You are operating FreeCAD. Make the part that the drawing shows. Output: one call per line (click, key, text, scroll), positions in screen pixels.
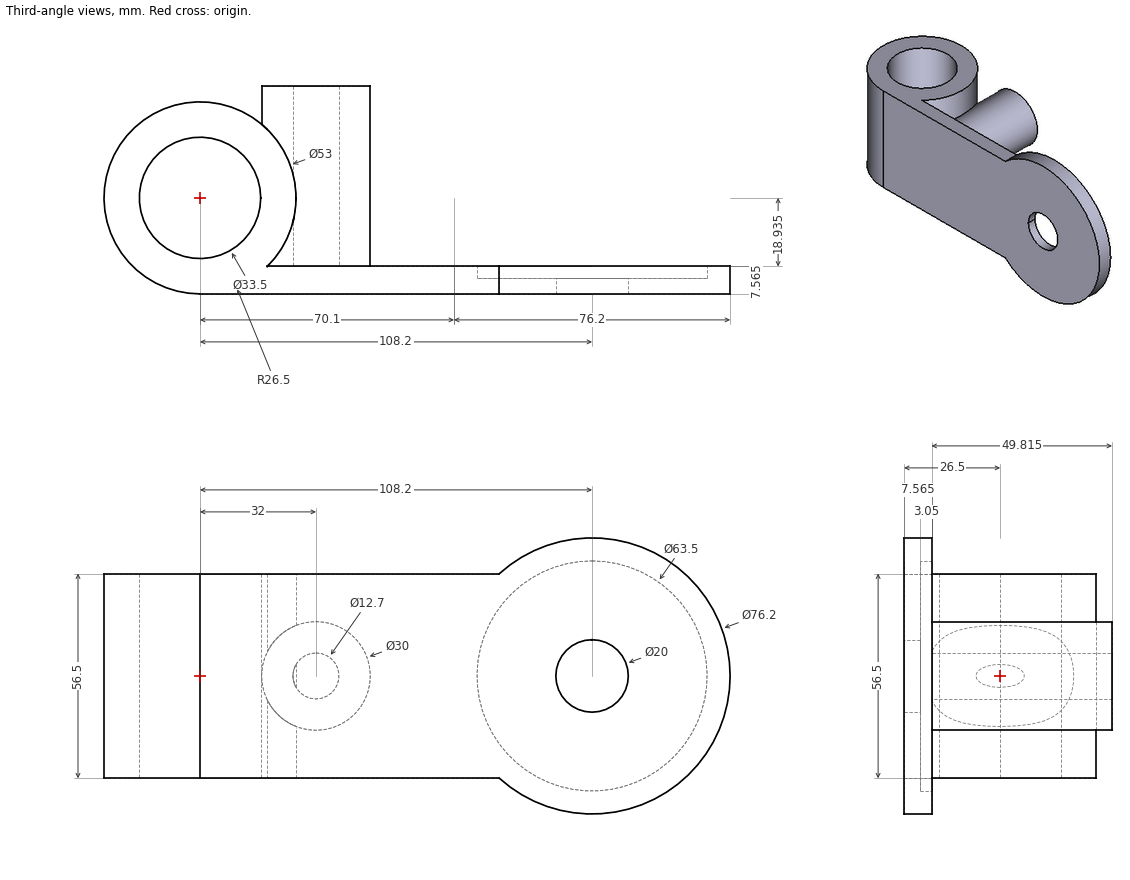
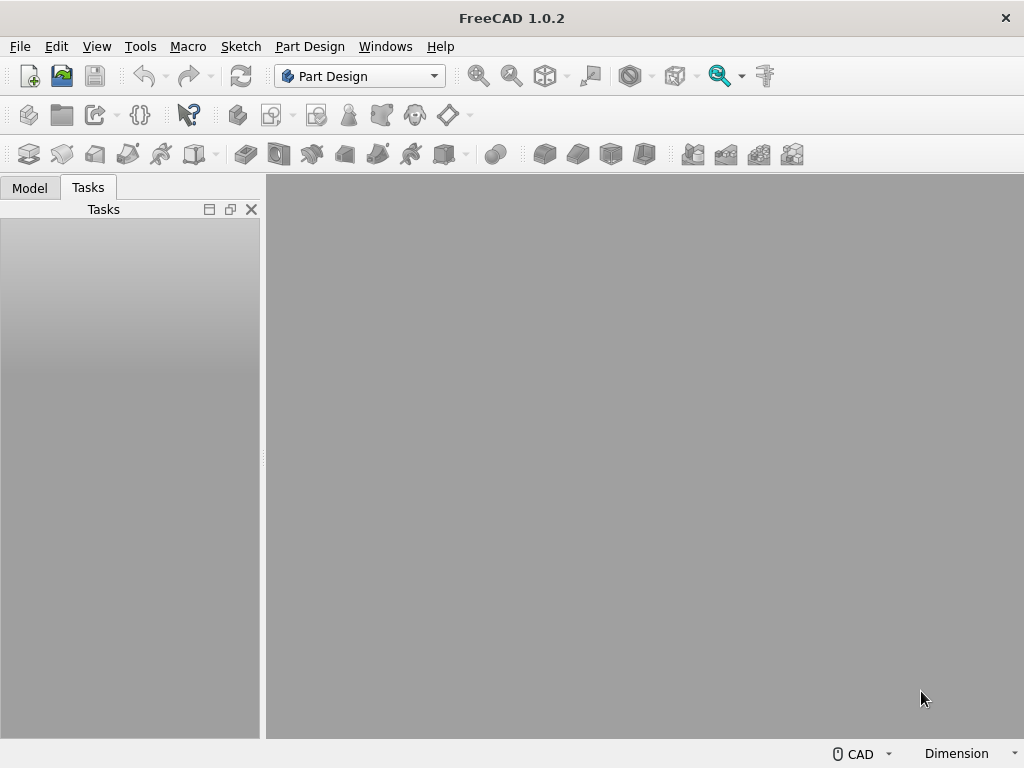
key(ctrl+n)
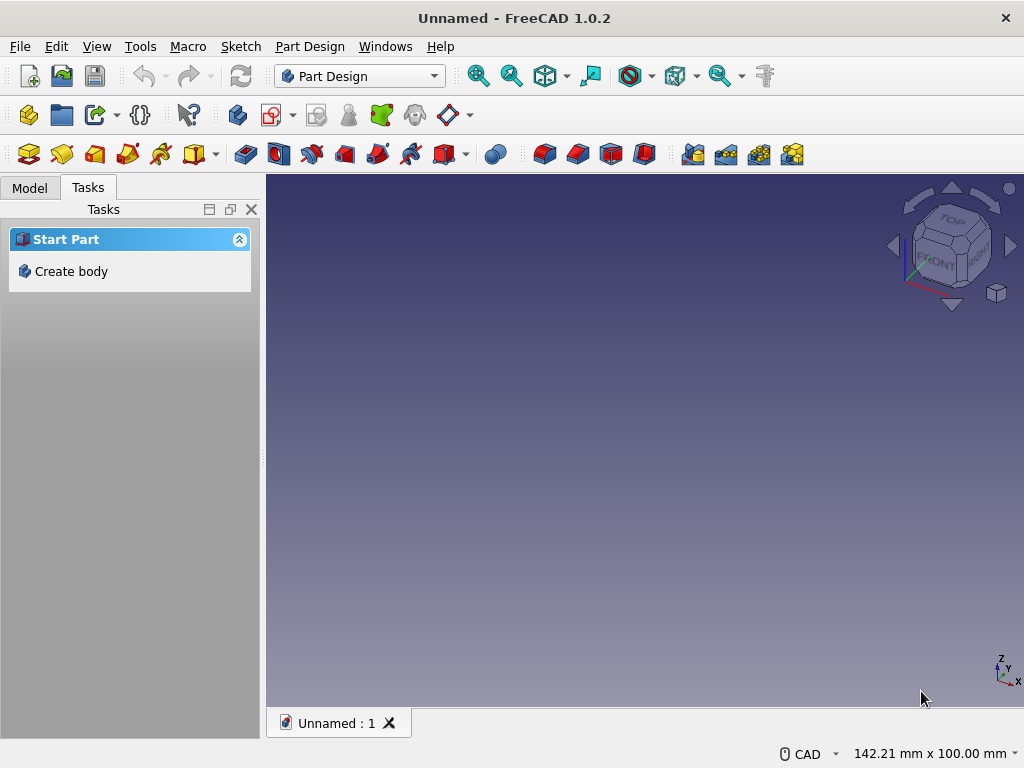
click(270, 116)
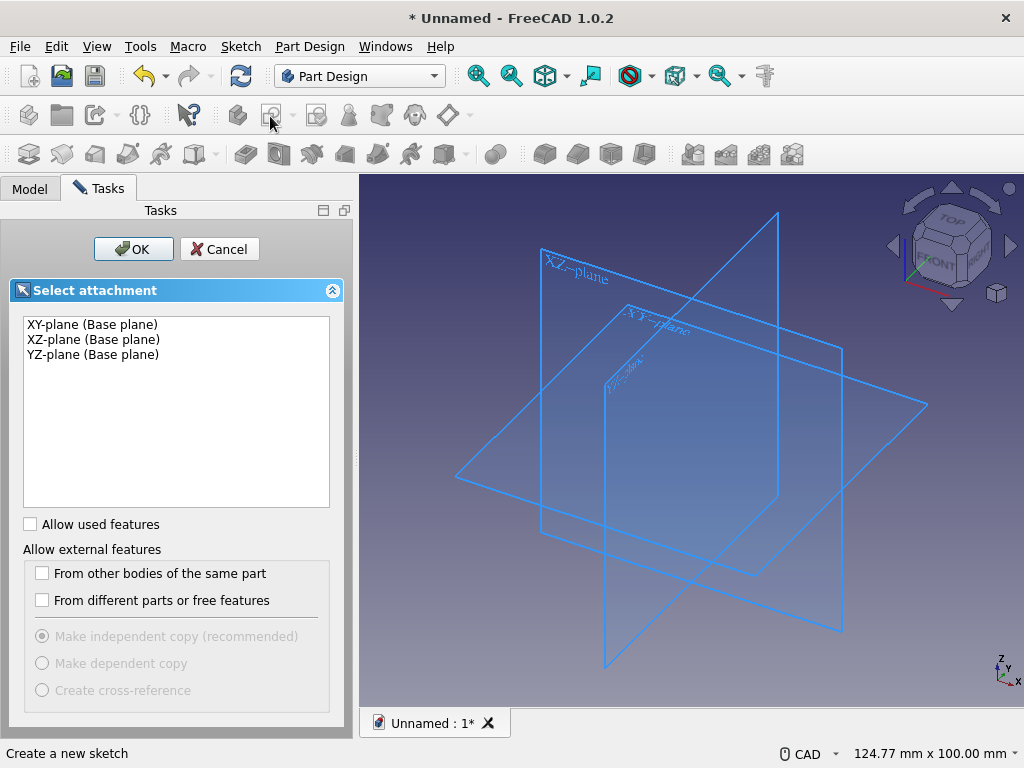
click(84, 324)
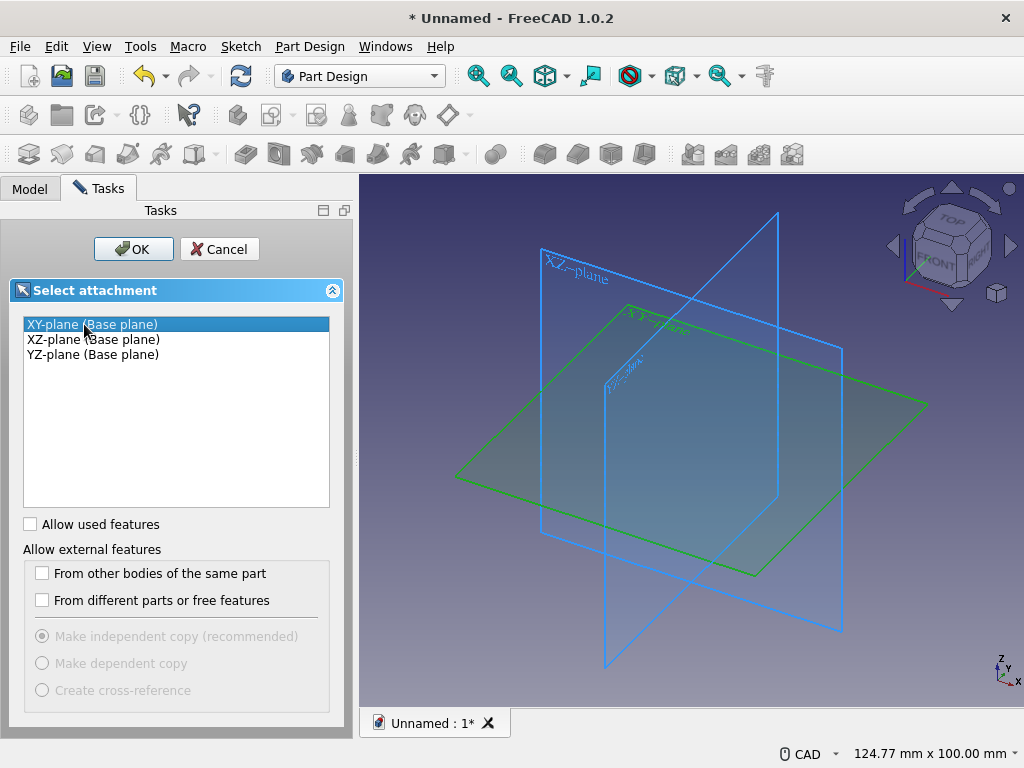
click(134, 249)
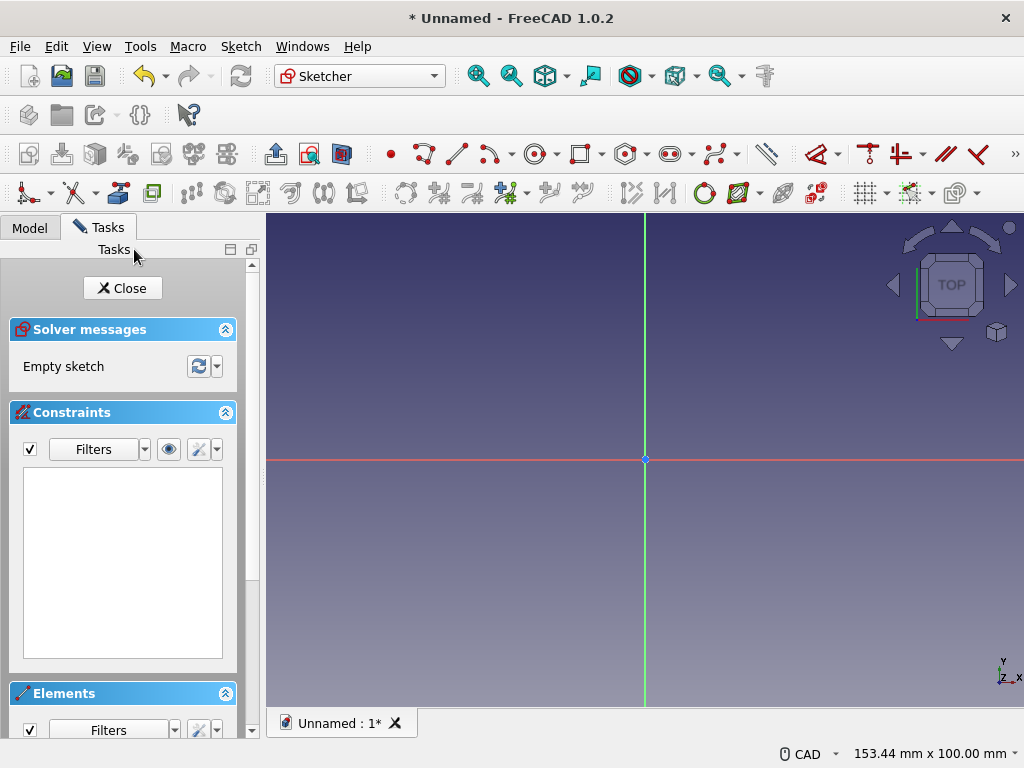
key(g)
key(c)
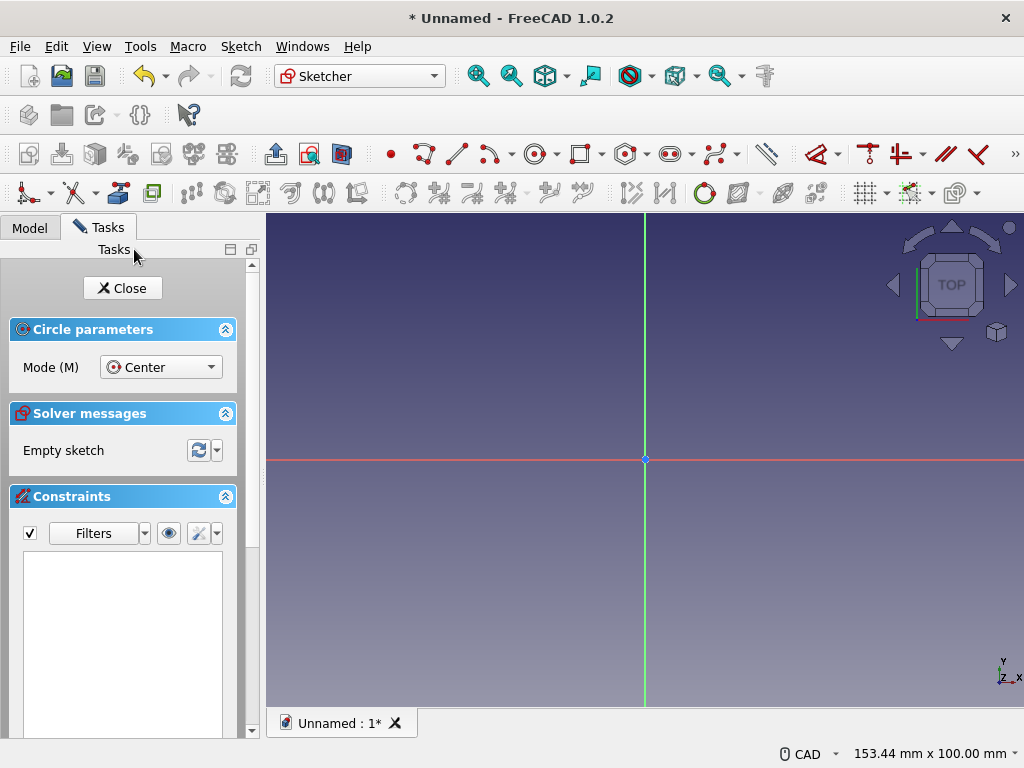
click(645, 460)
move(738, 367)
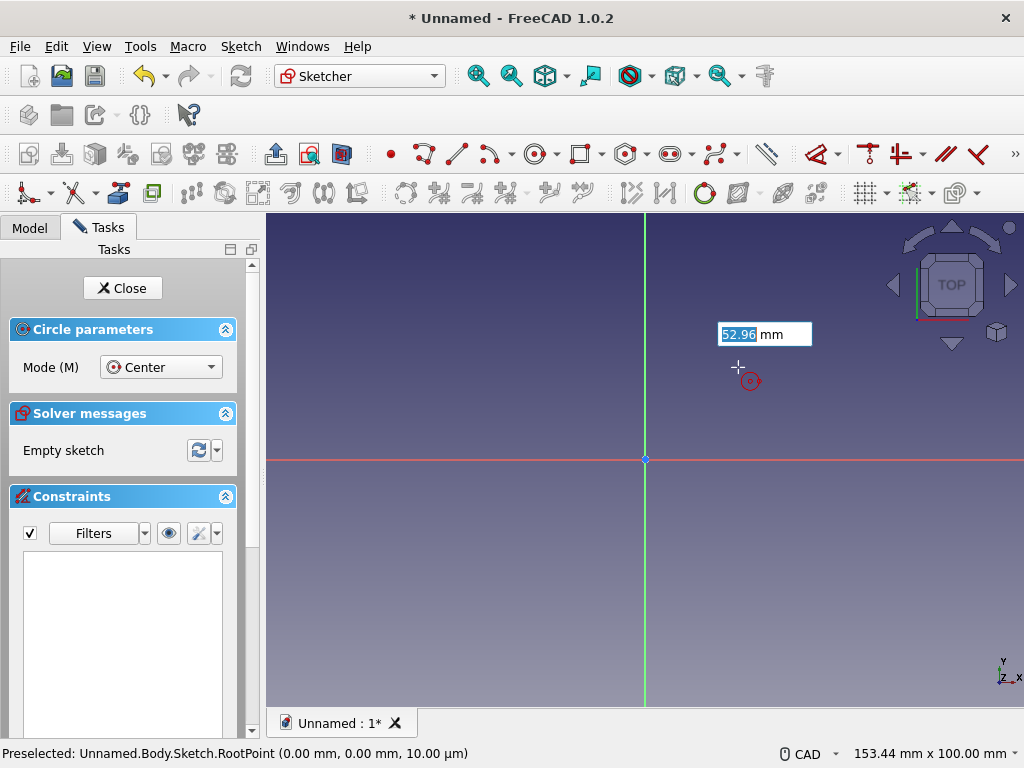
text(53)
key(Return)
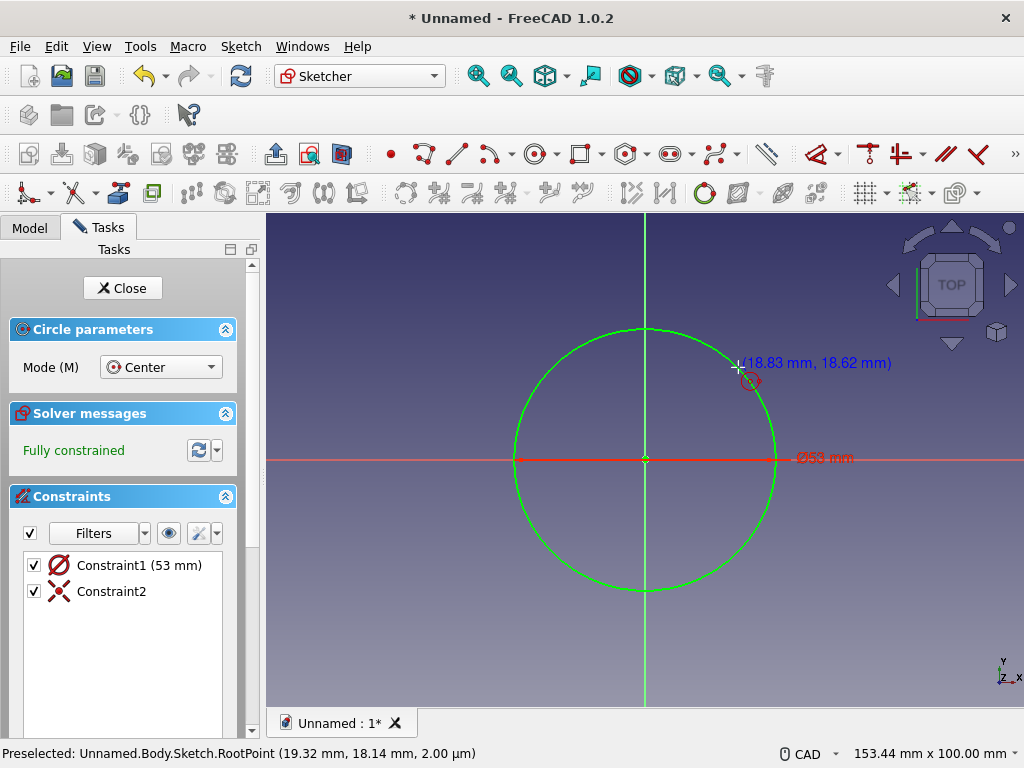
click(645, 460)
move(704, 401)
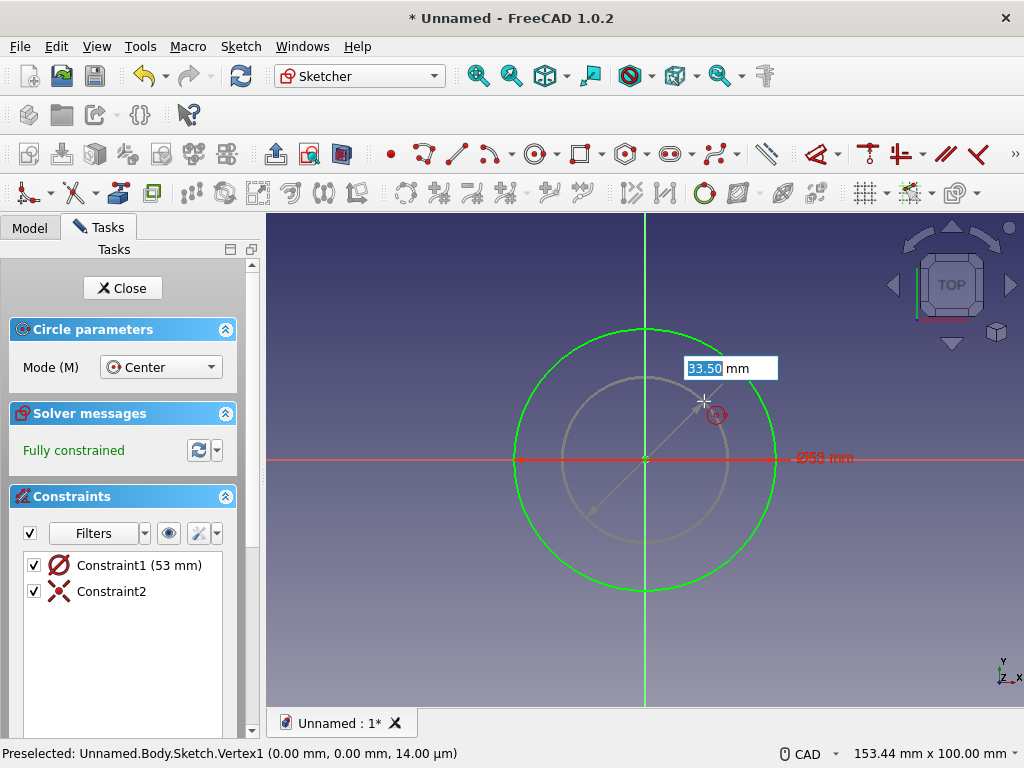
text(33.5)
key(Return)
key(Escape)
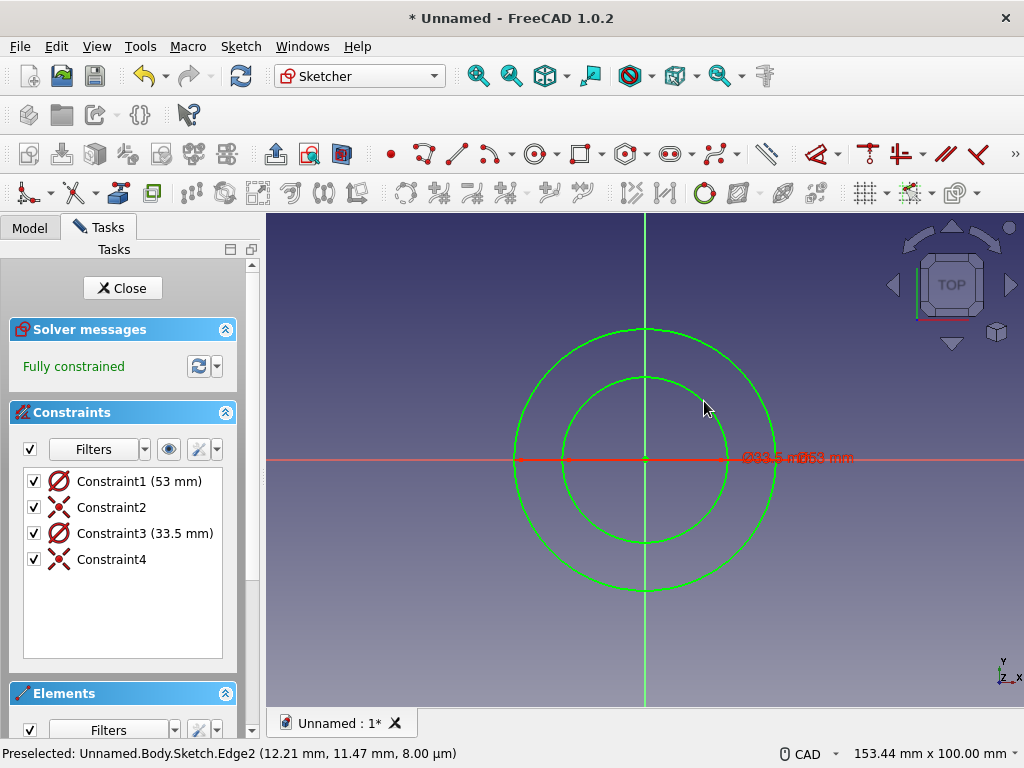
click(123, 288)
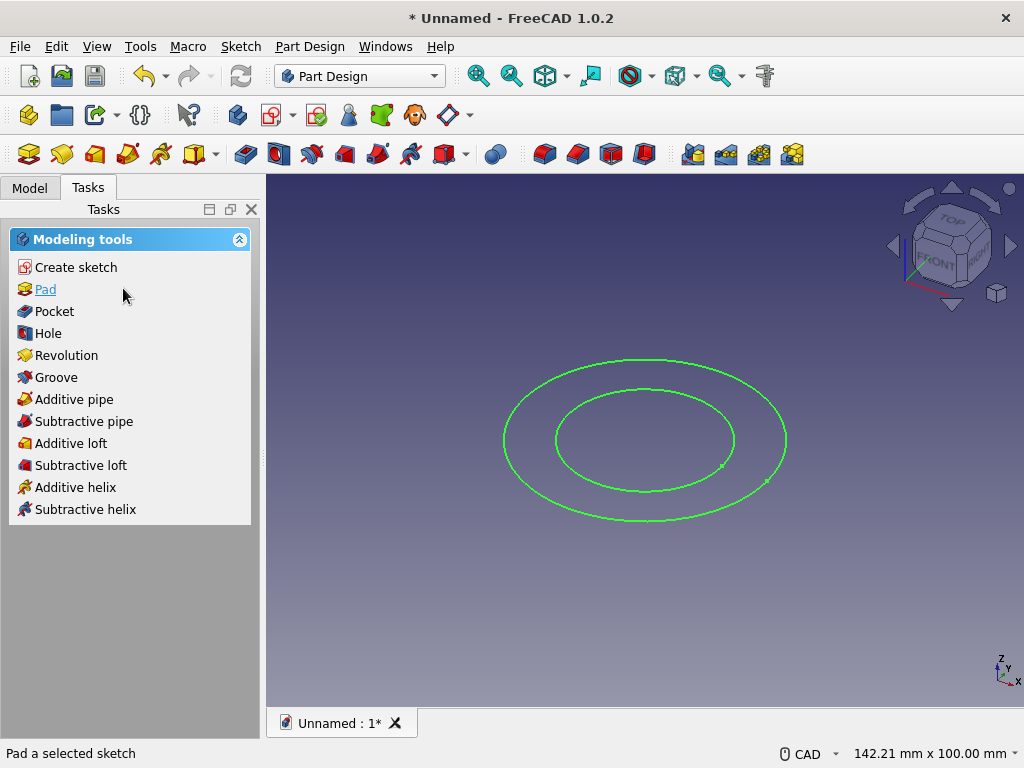
click(29, 154)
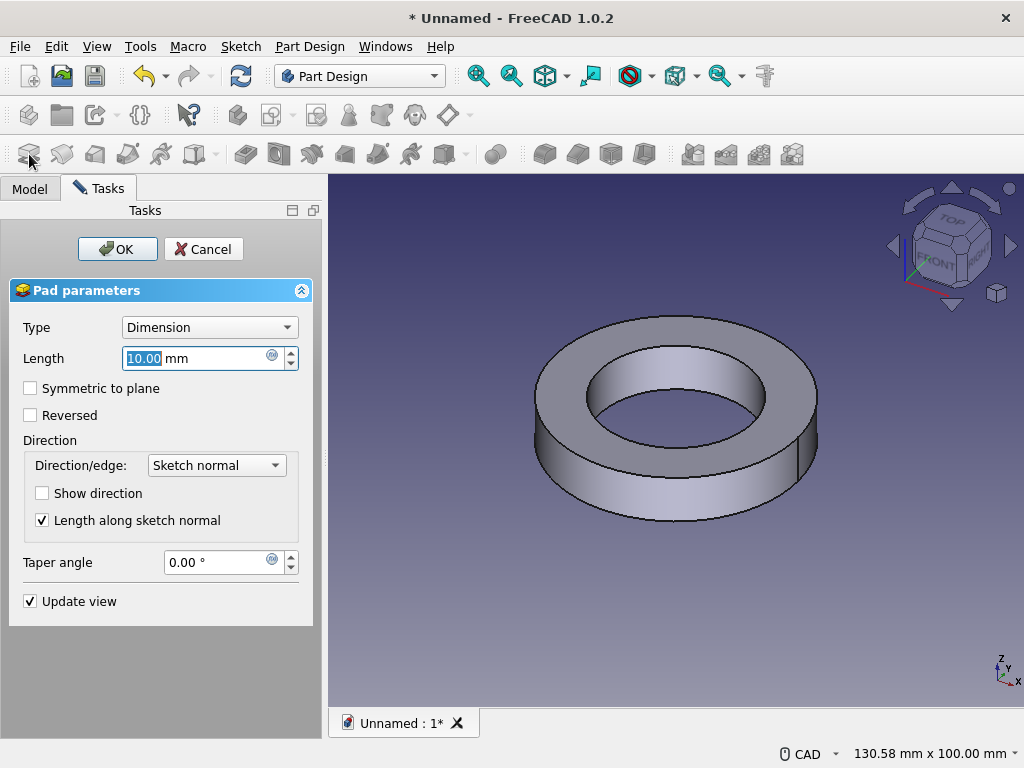
text(56.5)
key(Tab)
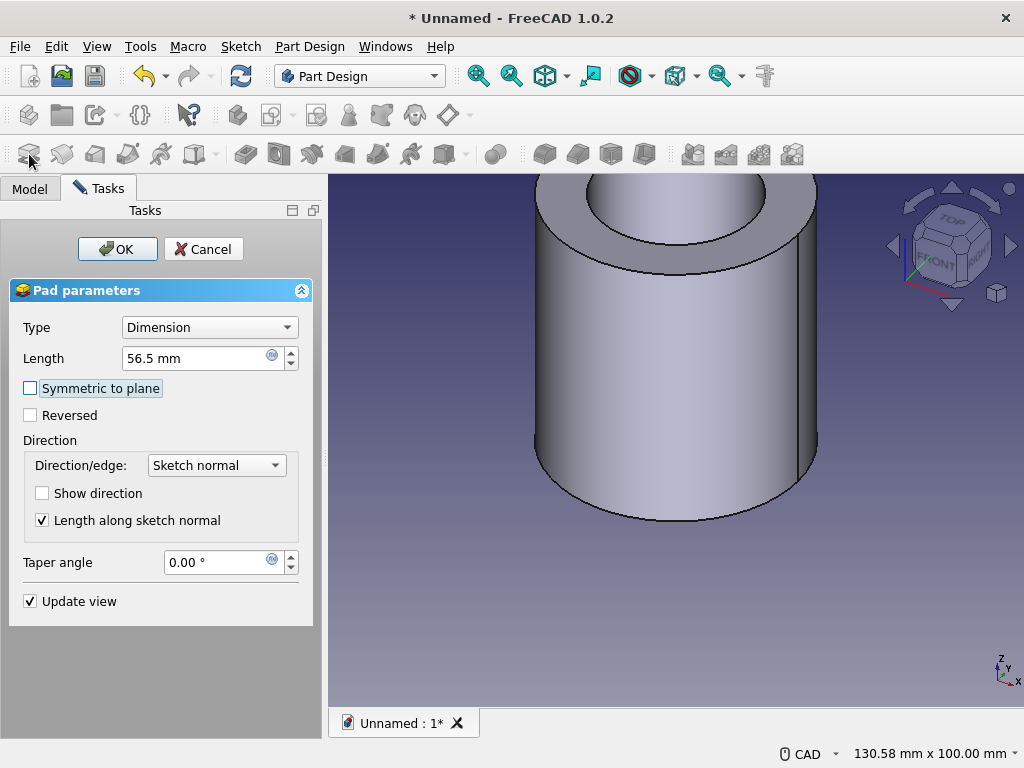
click(31, 388)